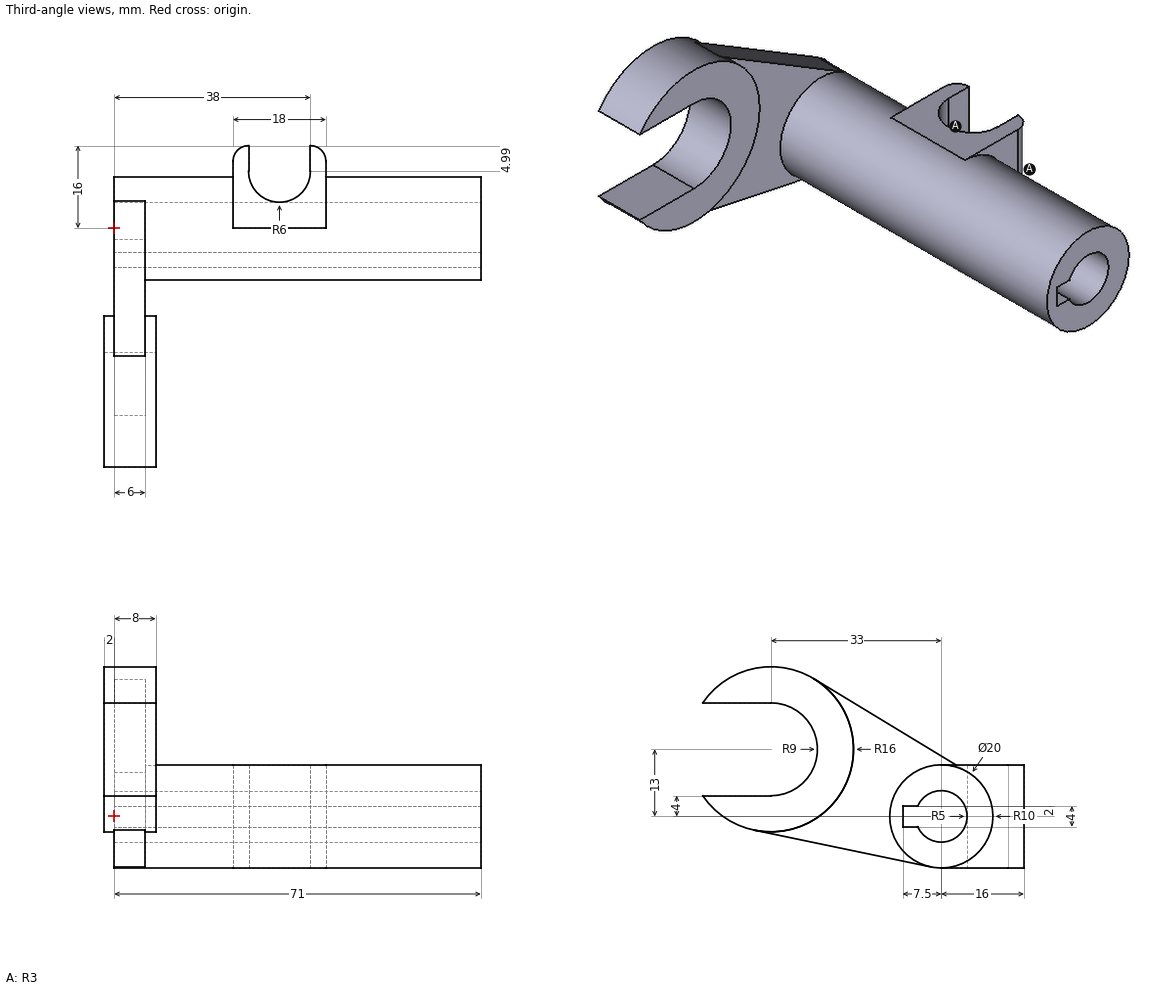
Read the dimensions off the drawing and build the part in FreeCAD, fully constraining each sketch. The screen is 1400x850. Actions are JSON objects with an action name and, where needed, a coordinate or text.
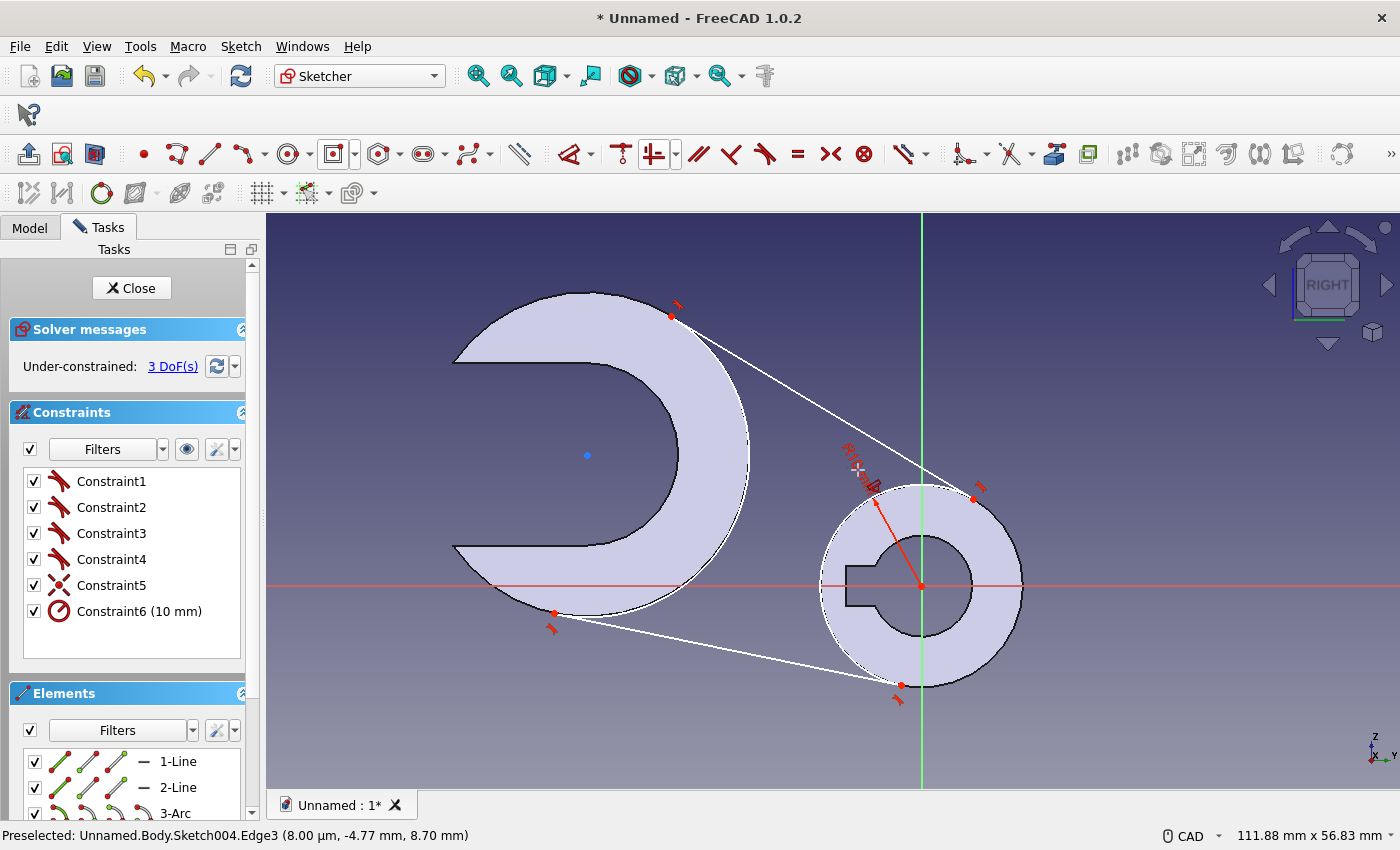
{"action": "left_click", "coordinate": [684, 586]}
{"action": "left_click", "coordinate": [703, 612]}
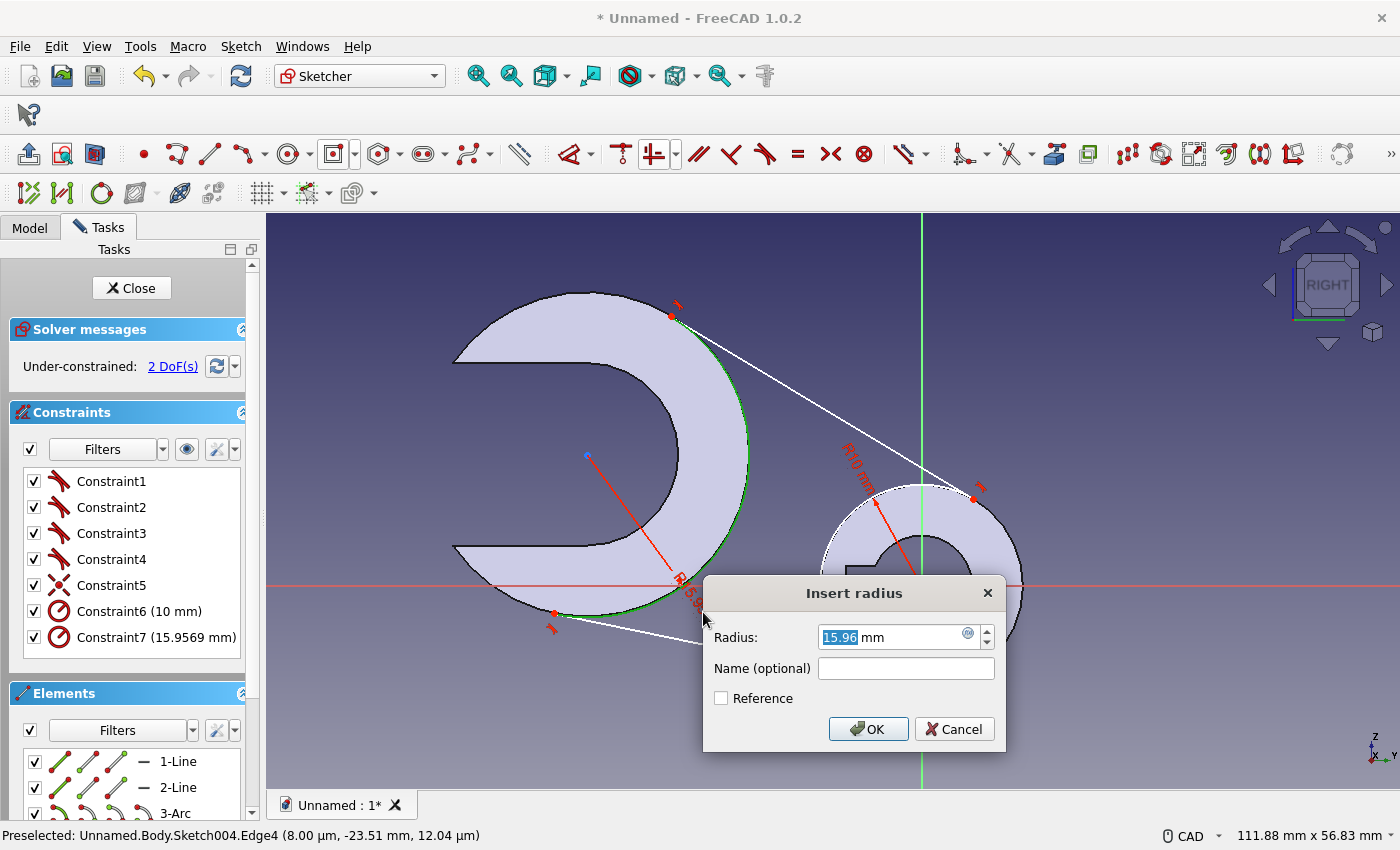
{"action": "type", "text": "16"}
{"action": "key", "text": "Return"}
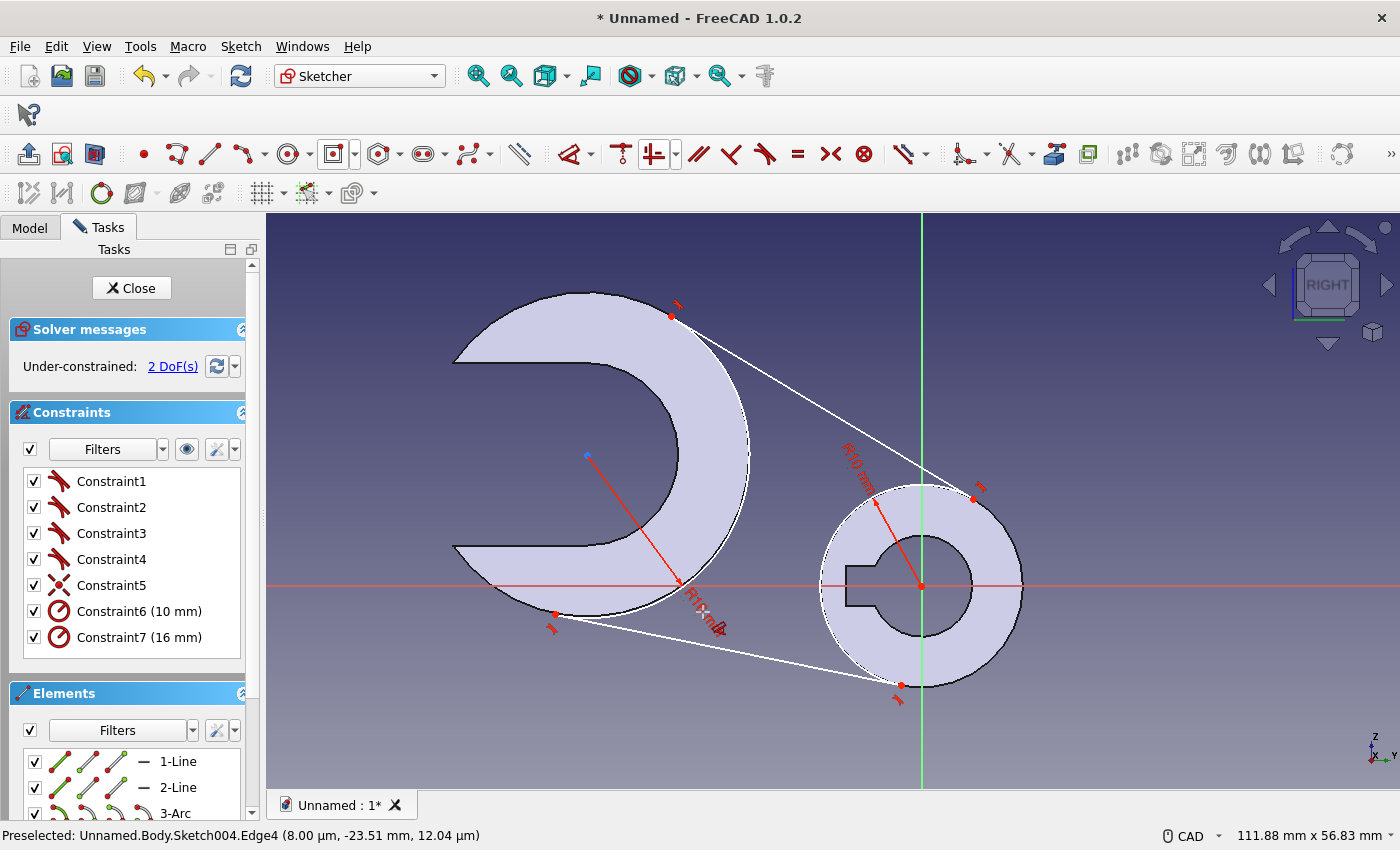
{"action": "left_click", "coordinate": [587, 456]}
{"action": "left_click", "coordinate": [871, 620]}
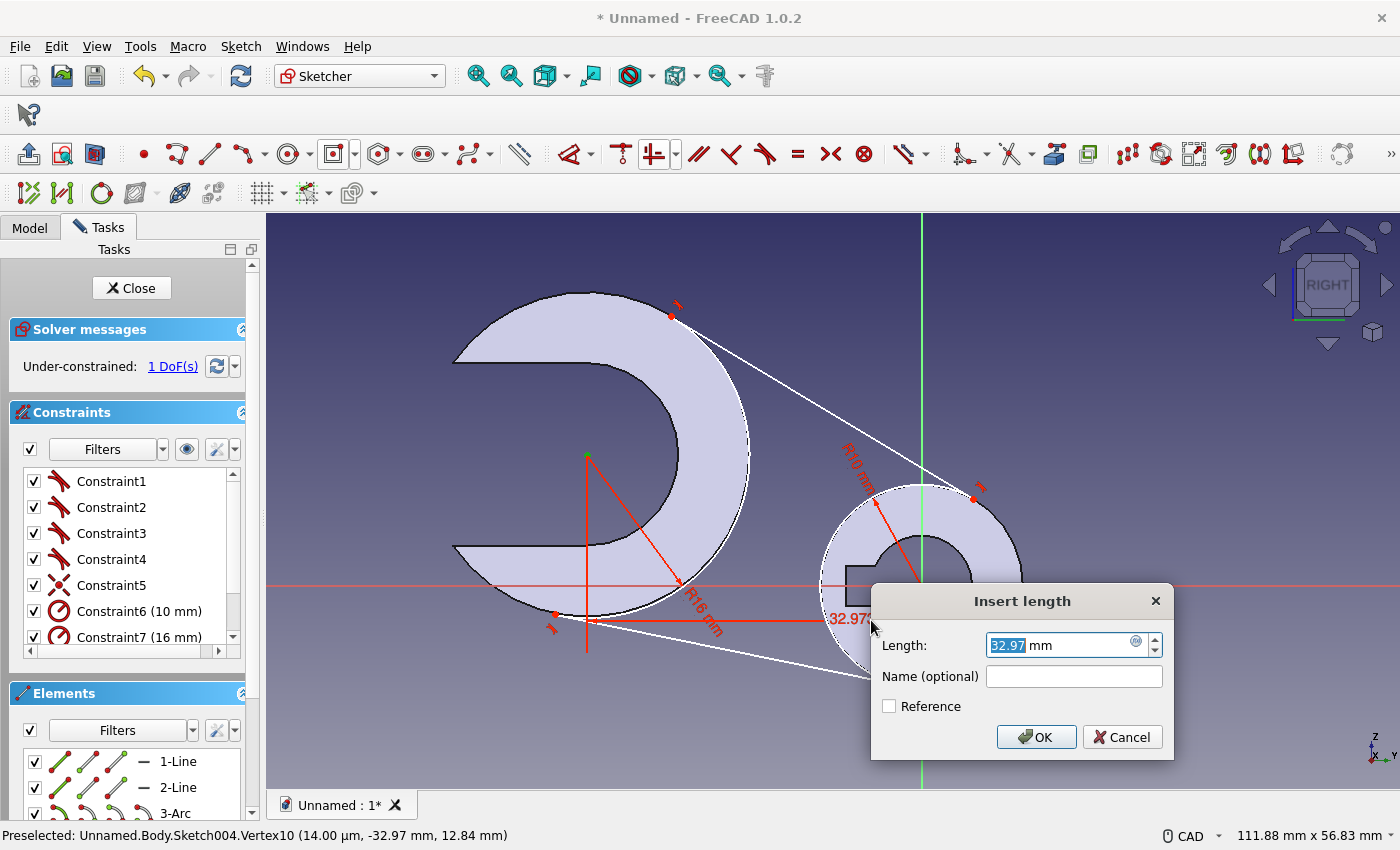
{"action": "type", "text": "33"}
{"action": "key", "text": "Return"}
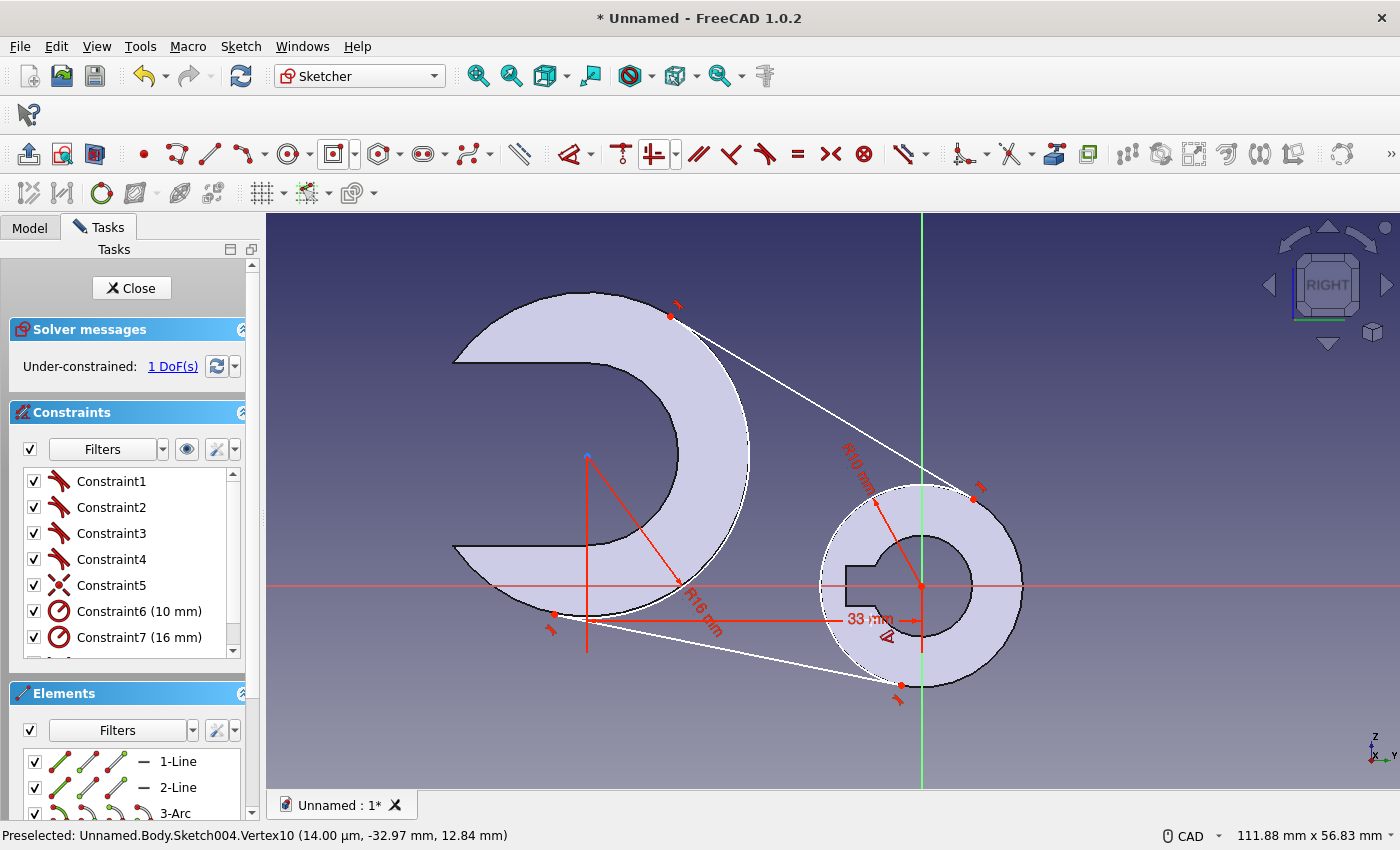
{"action": "left_click", "coordinate": [587, 456]}
{"action": "left_click", "coordinate": [553, 521]}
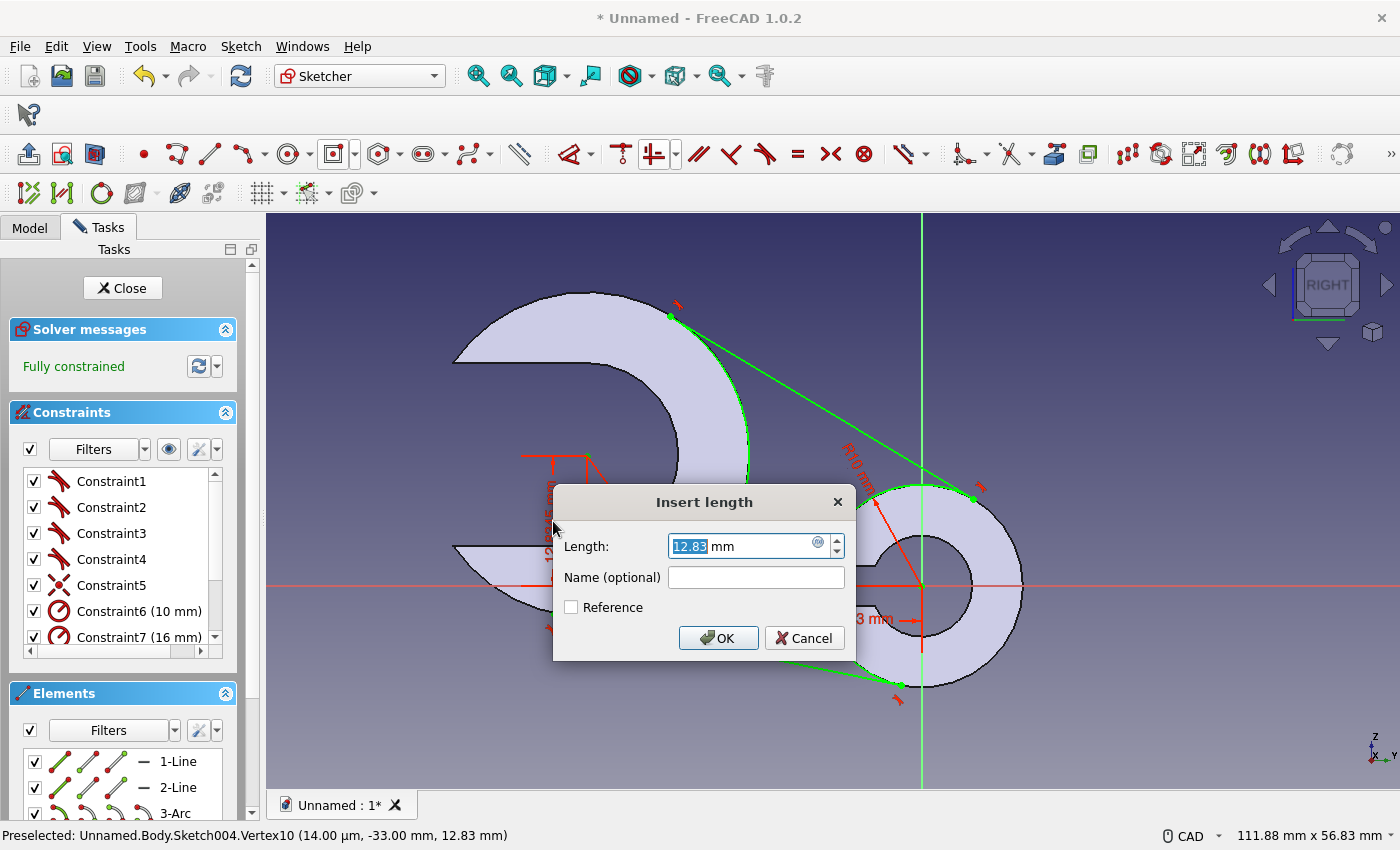
{"action": "type", "text": "13"}
{"action": "key", "text": "Return"}
{"action": "key", "text": "Escape"}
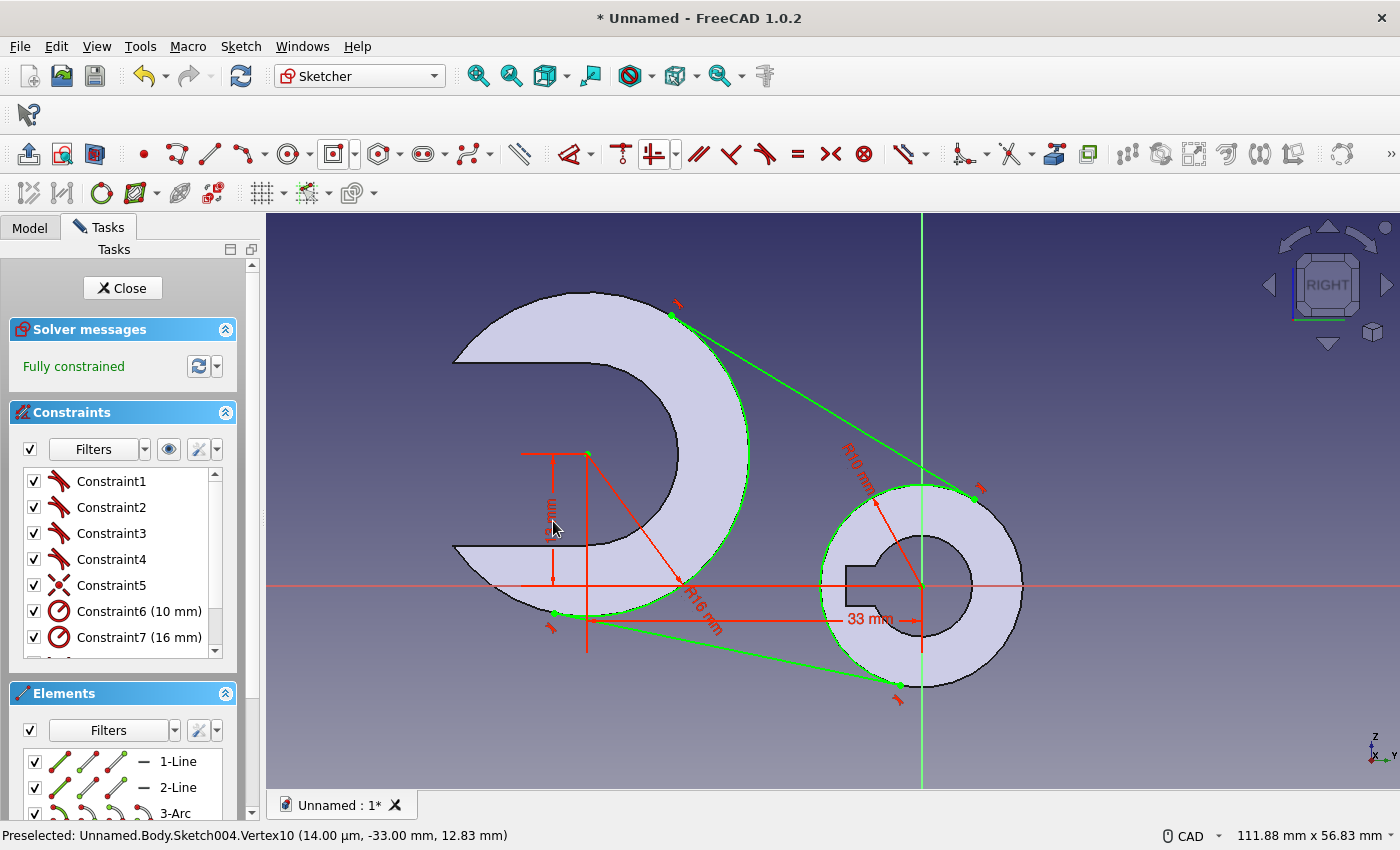
{"action": "left_click", "coordinate": [123, 288]}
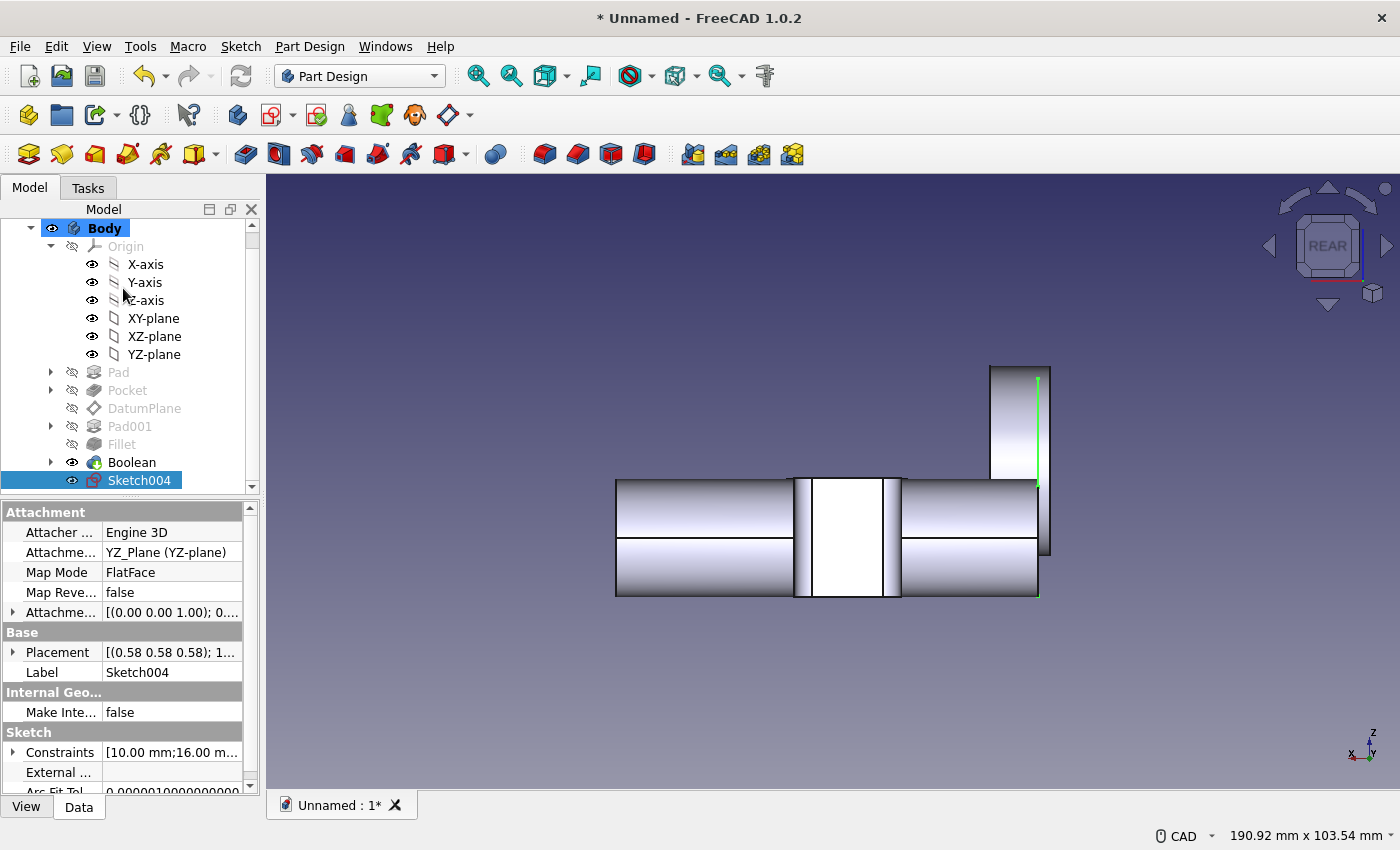
{"action": "left_click", "coordinate": [29, 154]}